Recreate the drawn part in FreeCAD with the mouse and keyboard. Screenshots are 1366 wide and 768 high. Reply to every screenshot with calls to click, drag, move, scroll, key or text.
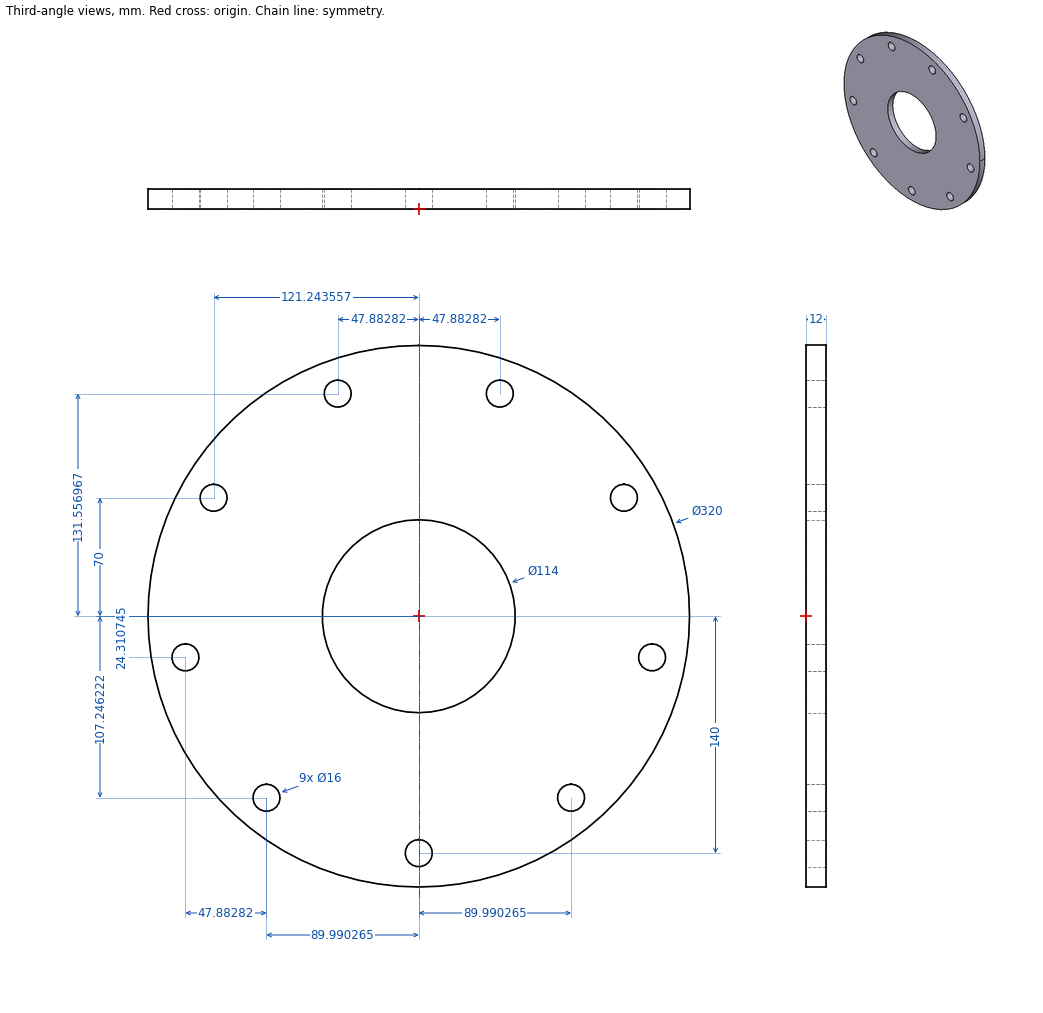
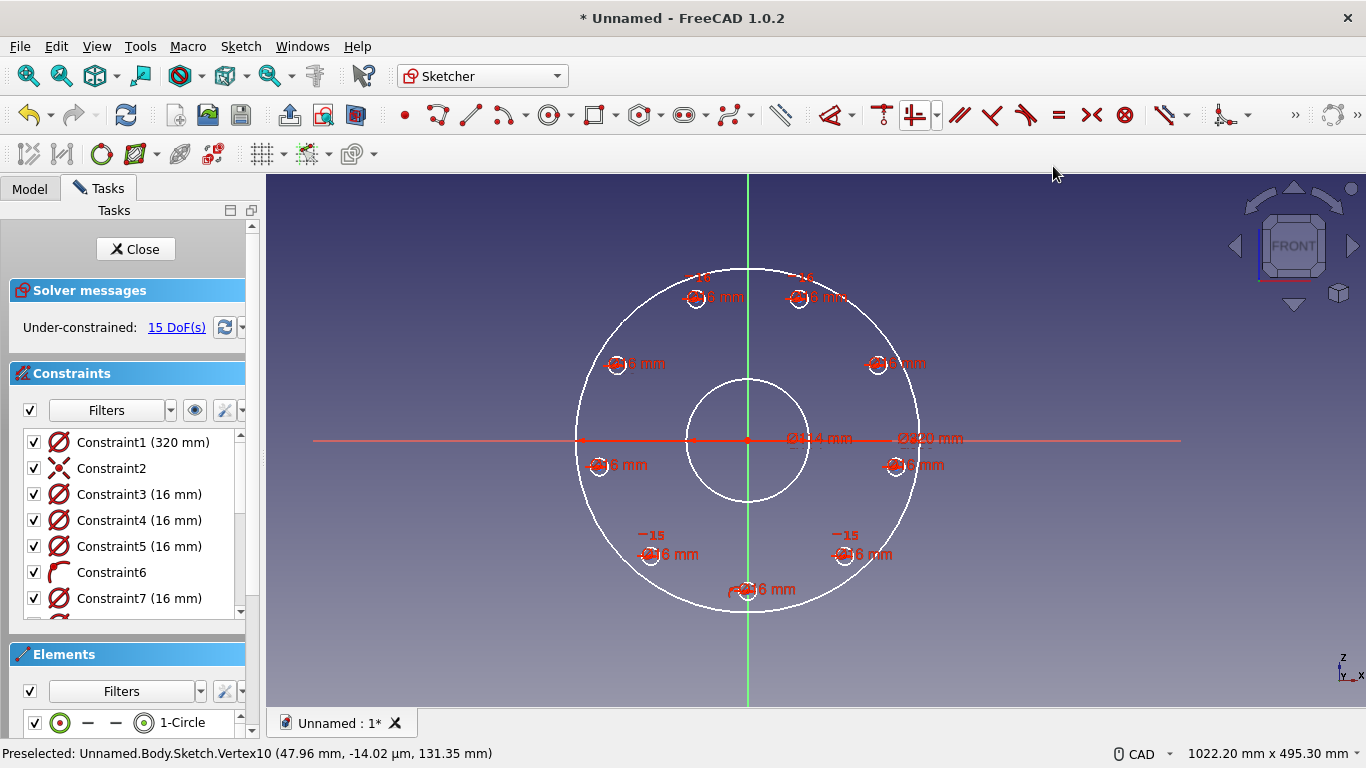
click(599, 467)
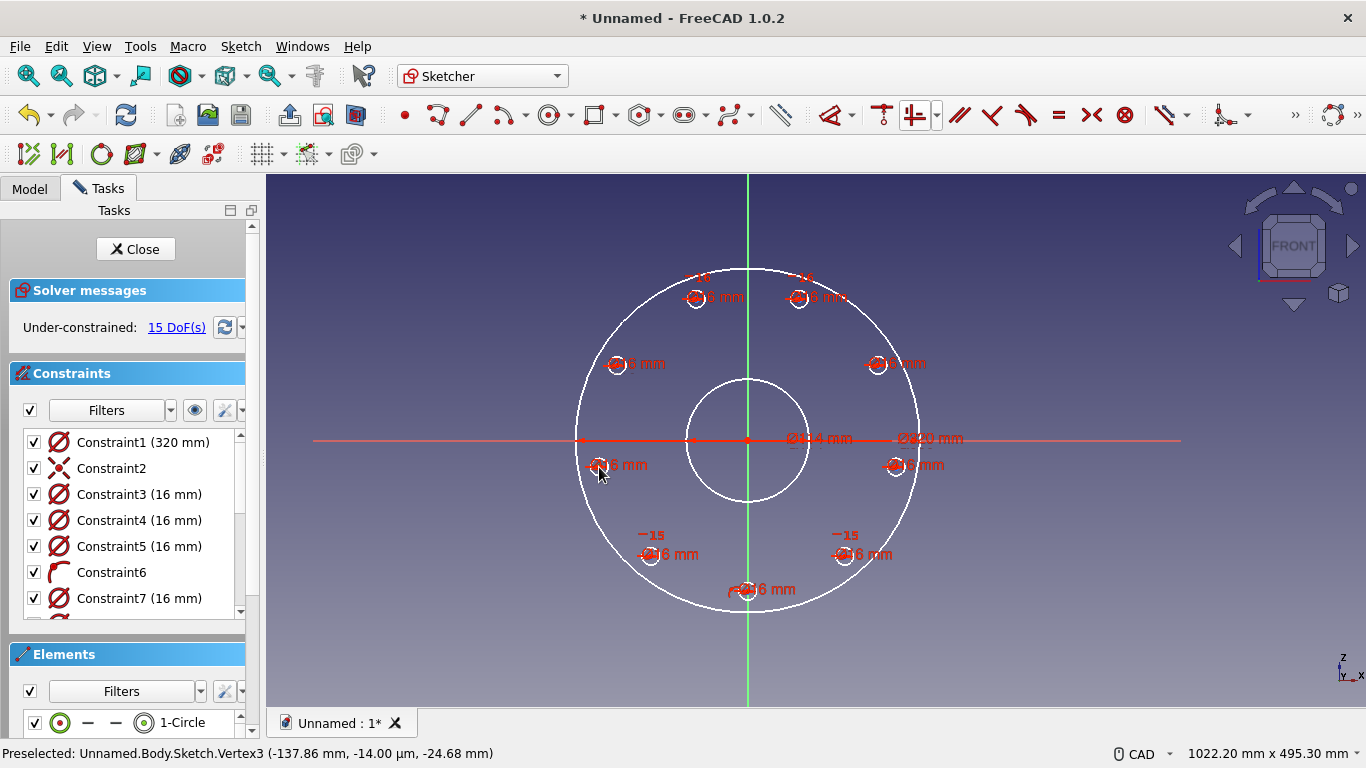
click(896, 467)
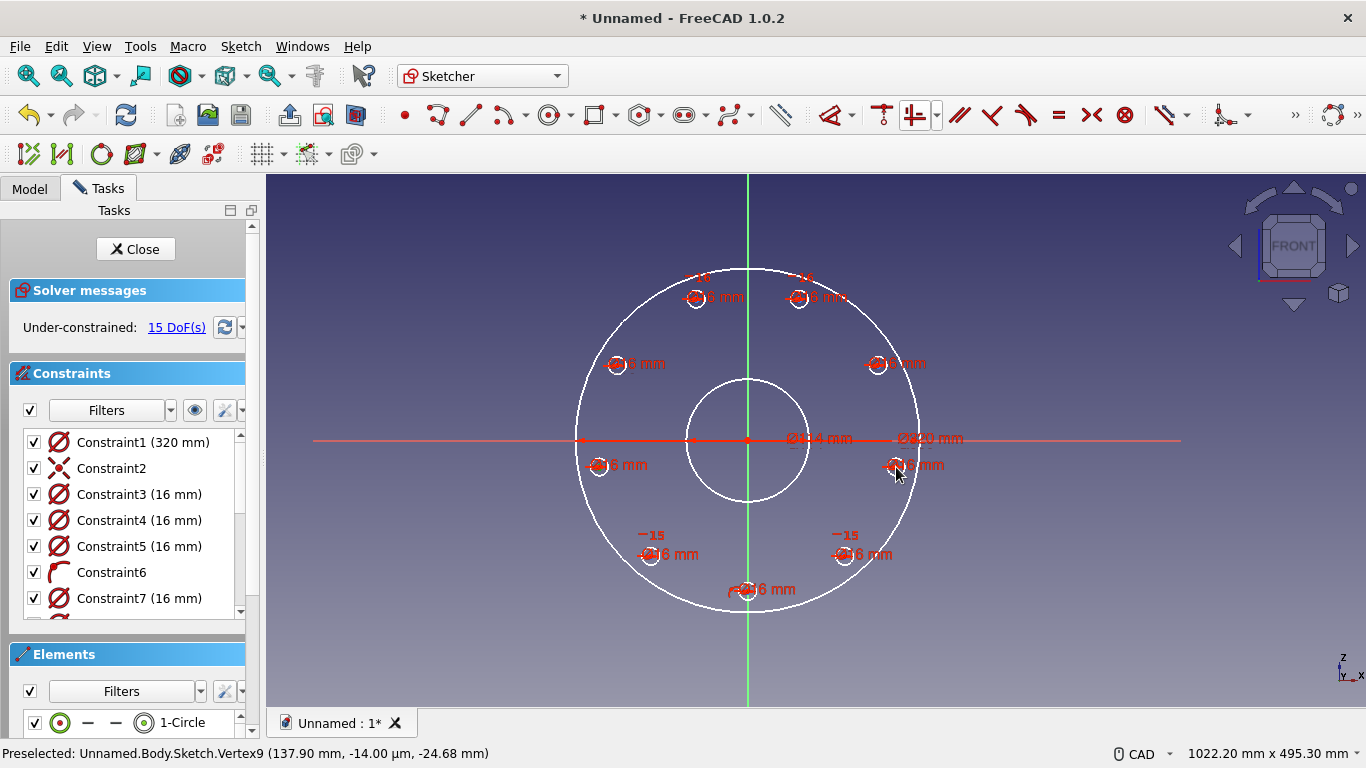
click(748, 645)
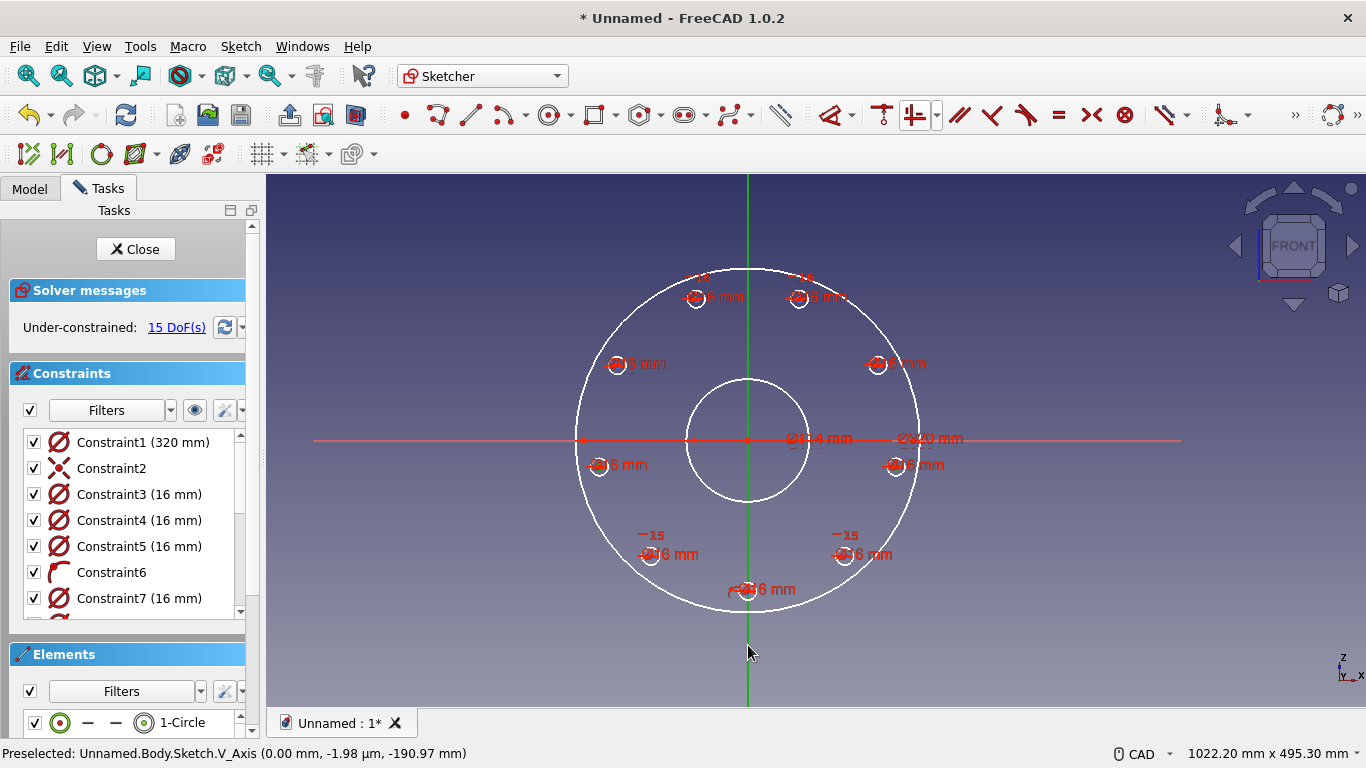
click(1092, 116)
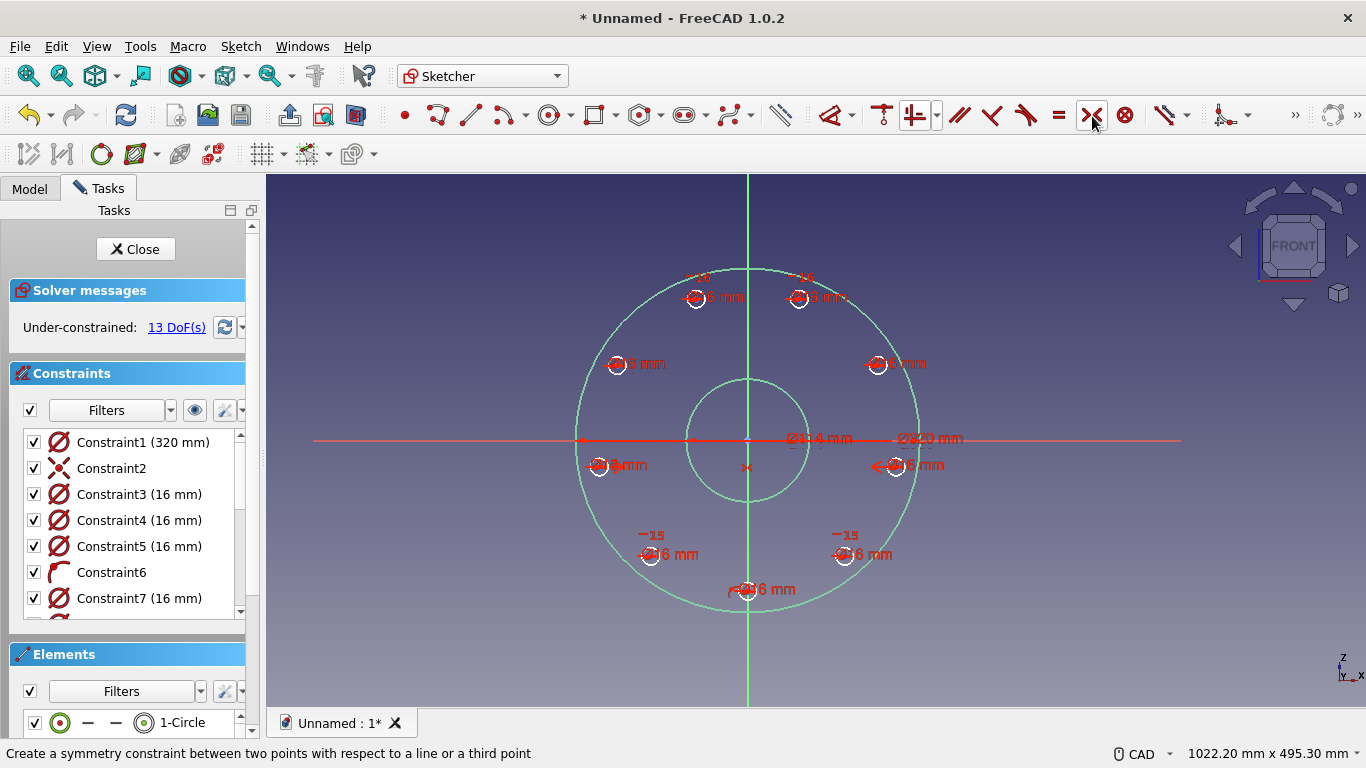
click(617, 366)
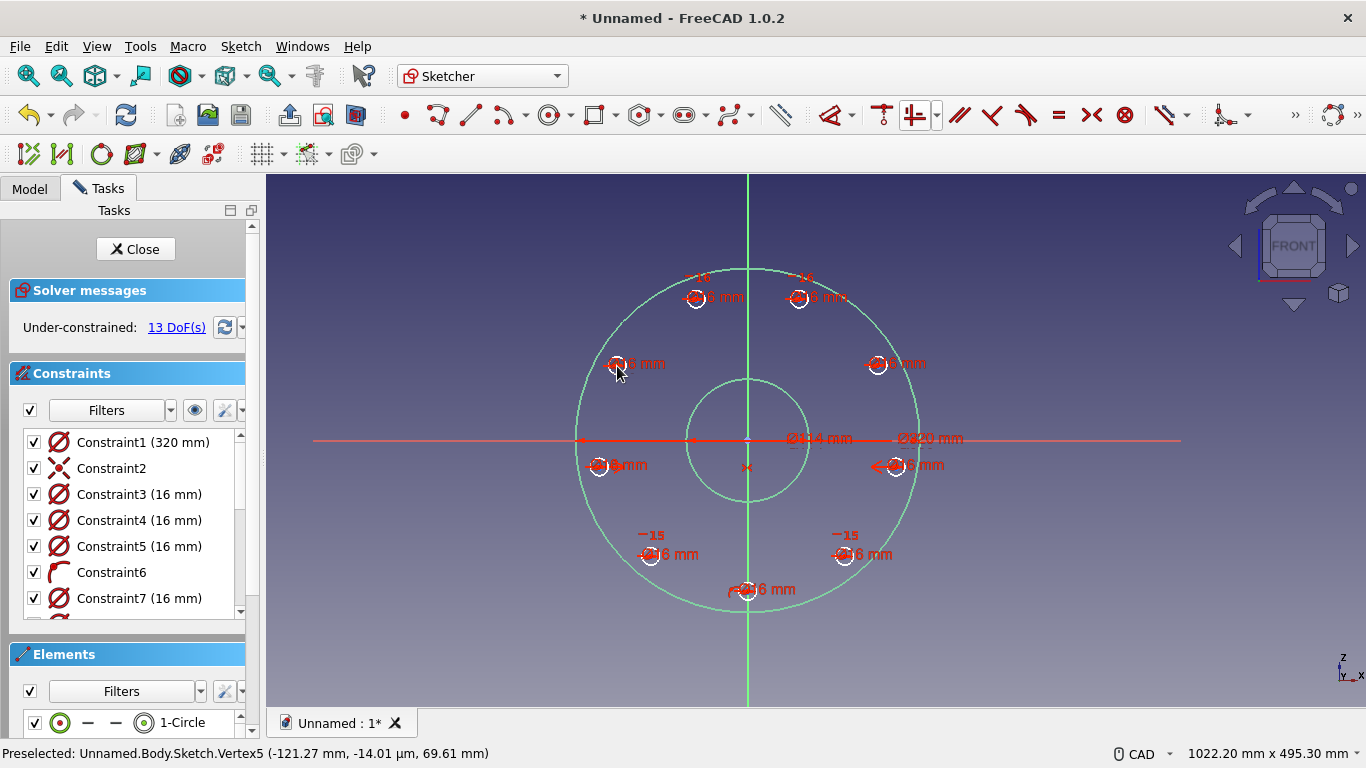
click(878, 365)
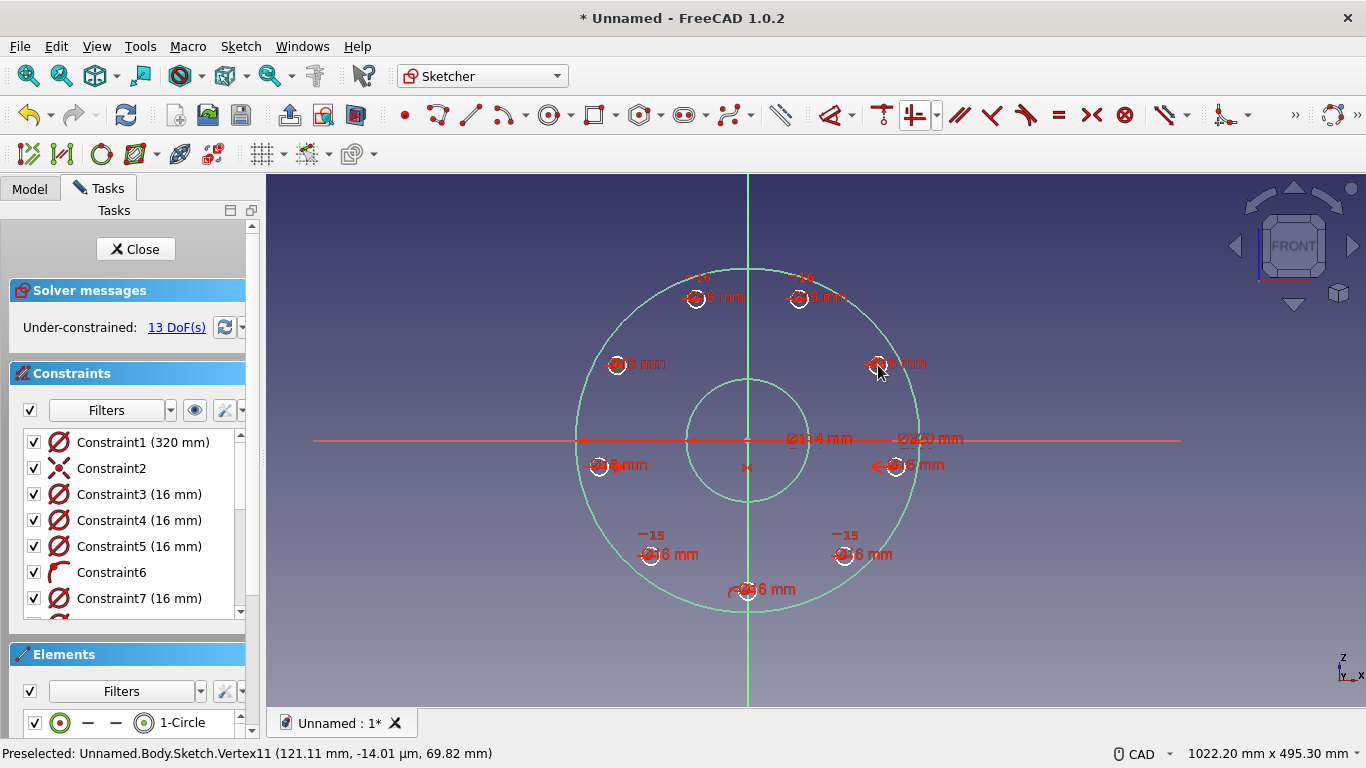
click(748, 645)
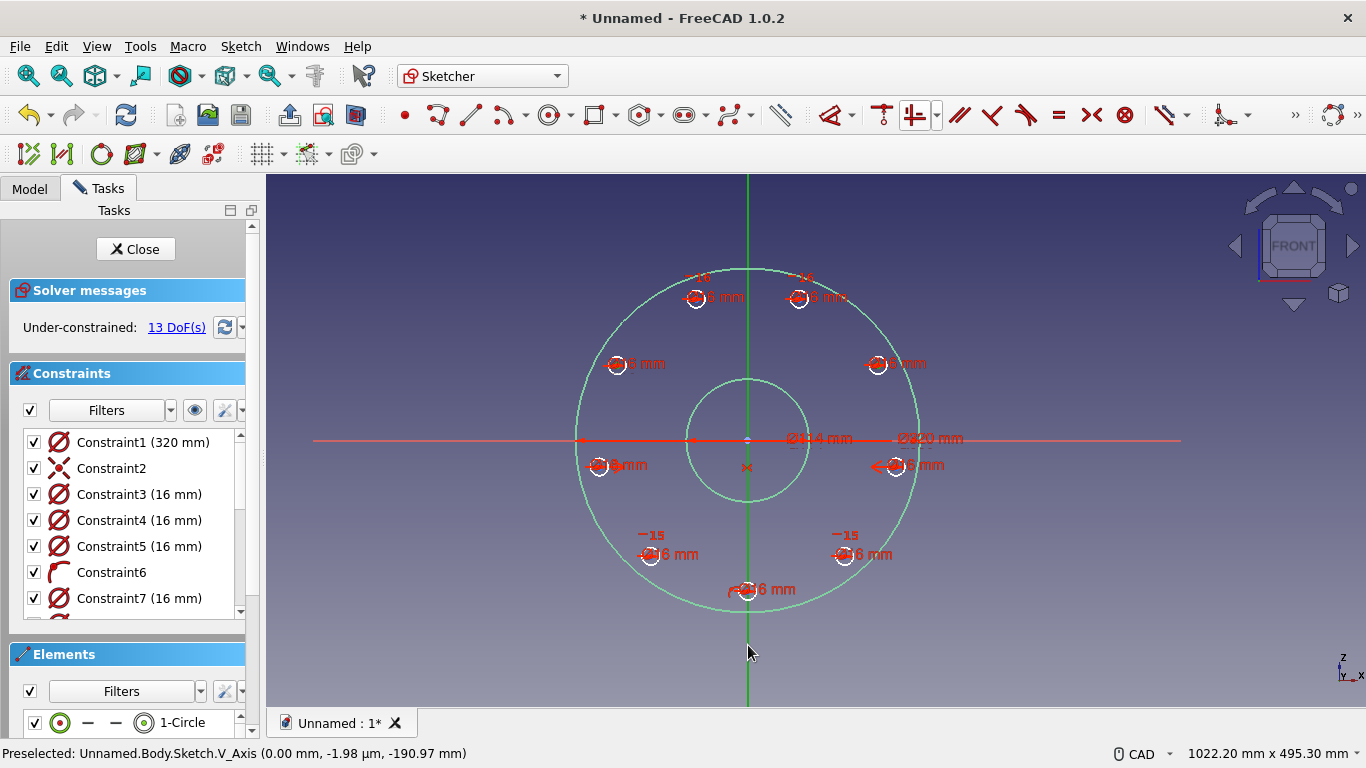
click(1092, 116)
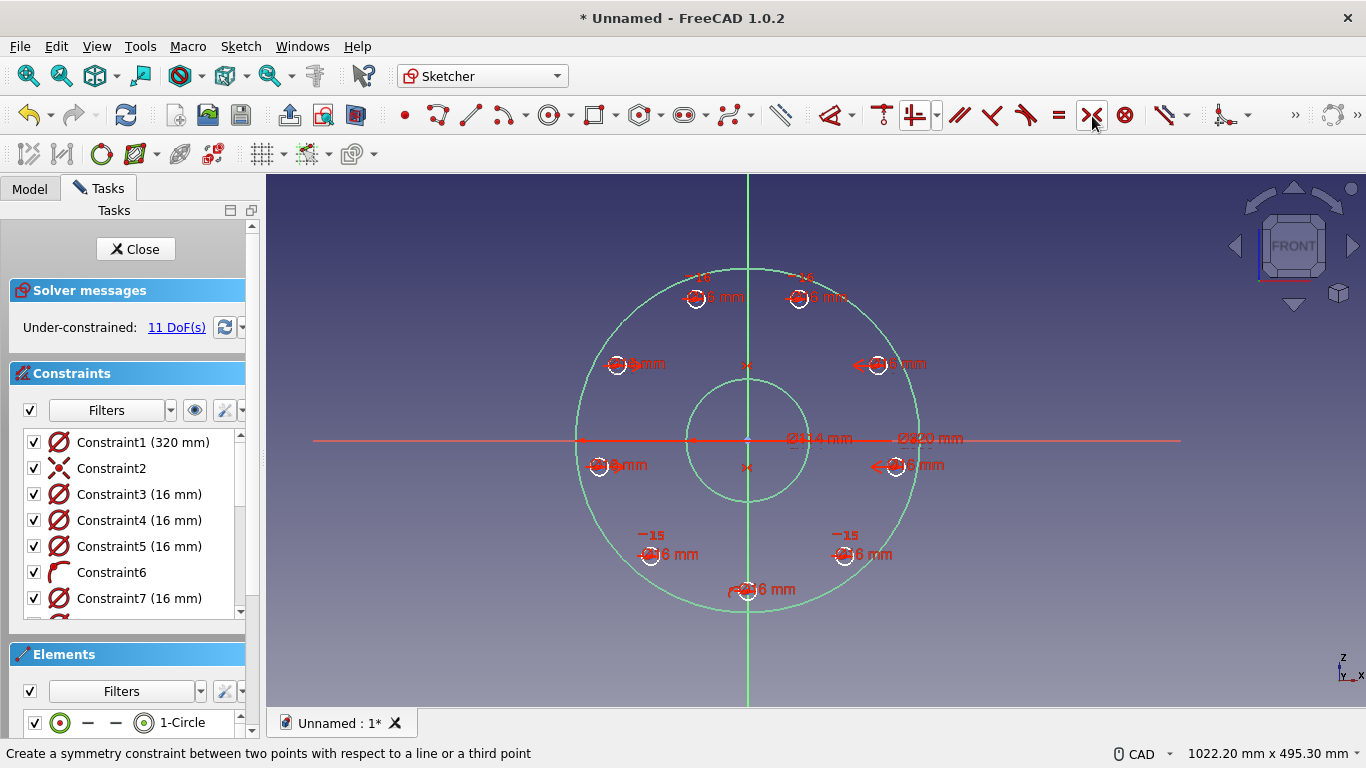
click(830, 116)